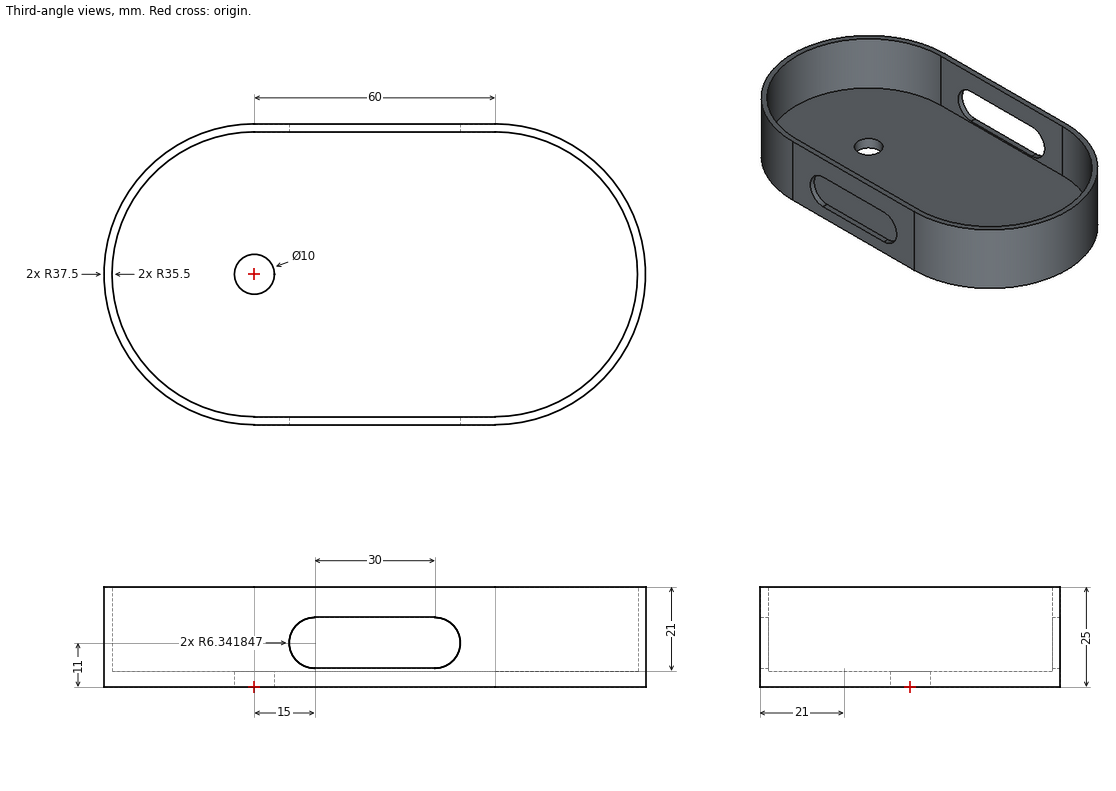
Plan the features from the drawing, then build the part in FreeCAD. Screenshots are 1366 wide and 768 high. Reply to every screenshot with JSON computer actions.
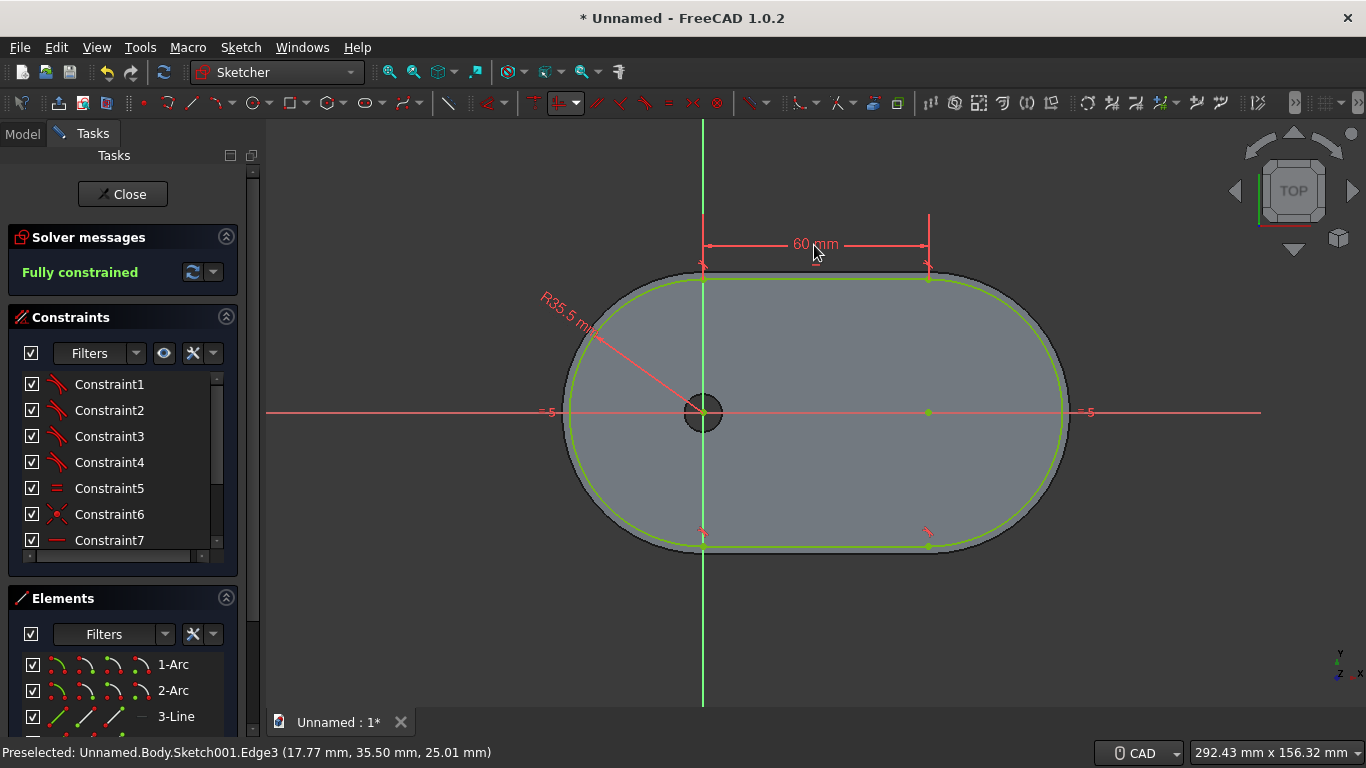
{"action": "left_click", "coordinate": [123, 194]}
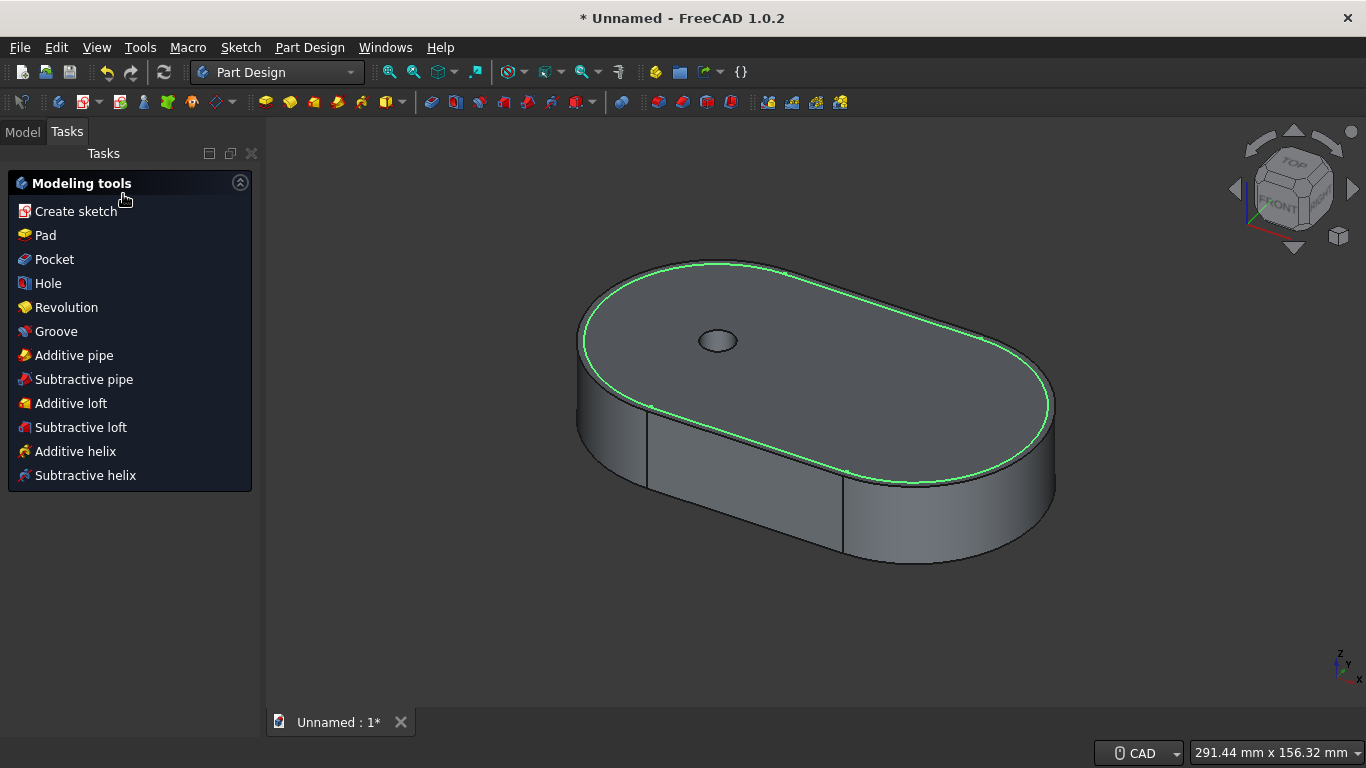
{"action": "left_click", "coordinate": [432, 102]}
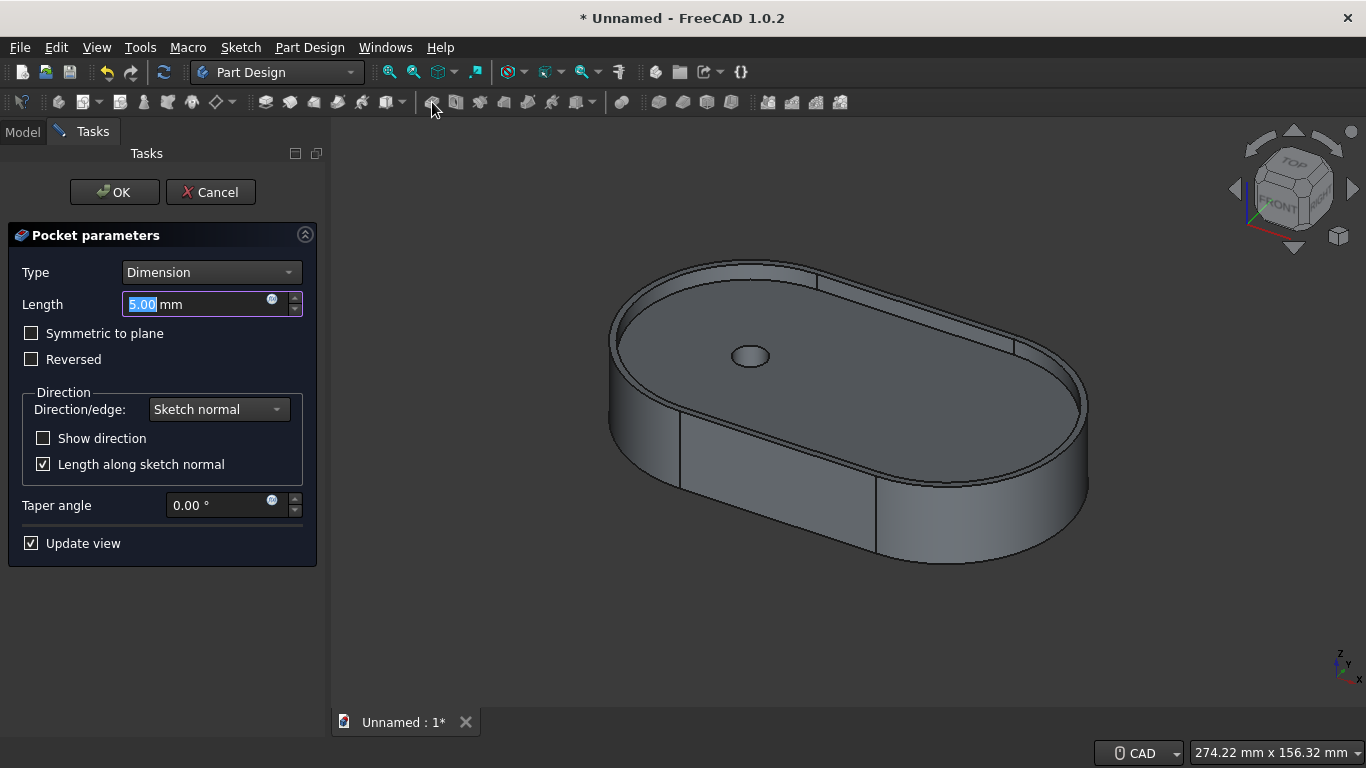
{"action": "type", "text": "21"}
{"action": "key", "text": "Tab"}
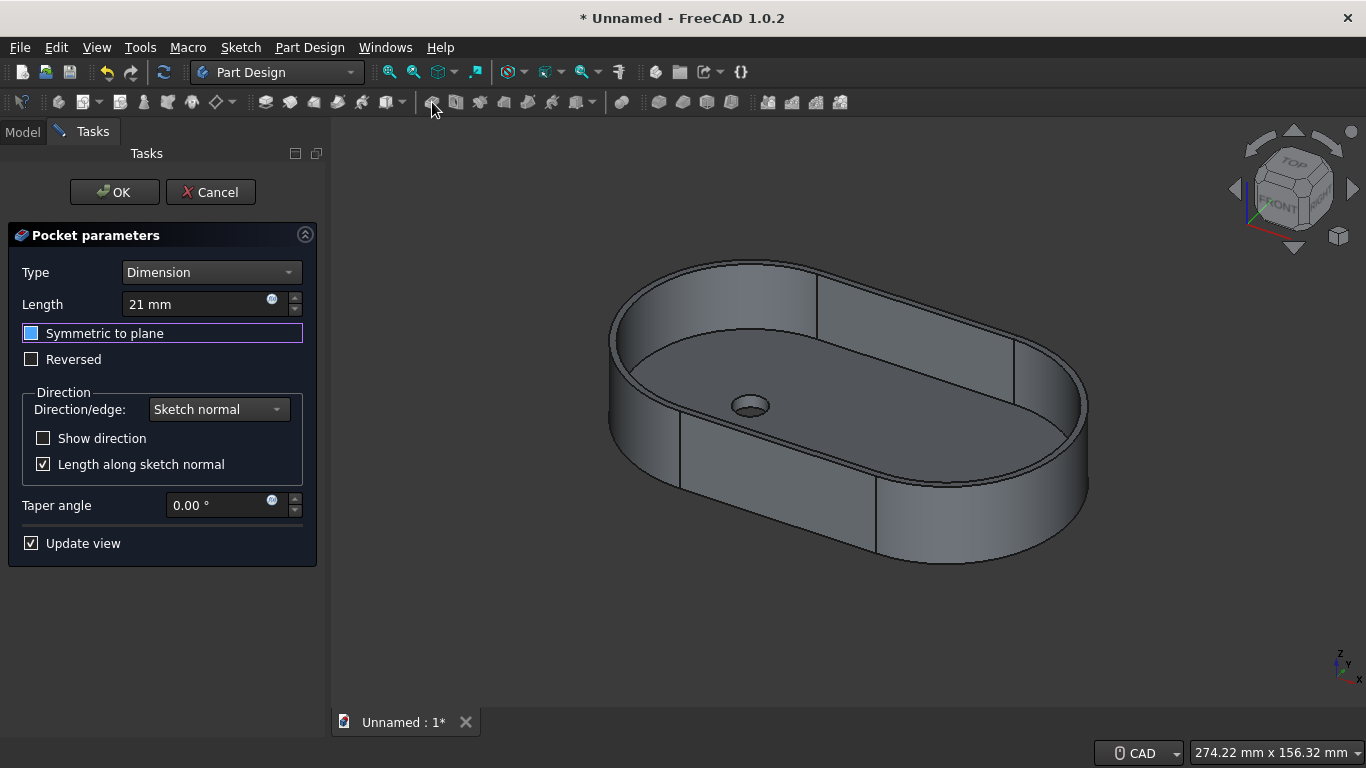
{"action": "left_click", "coordinate": [115, 192]}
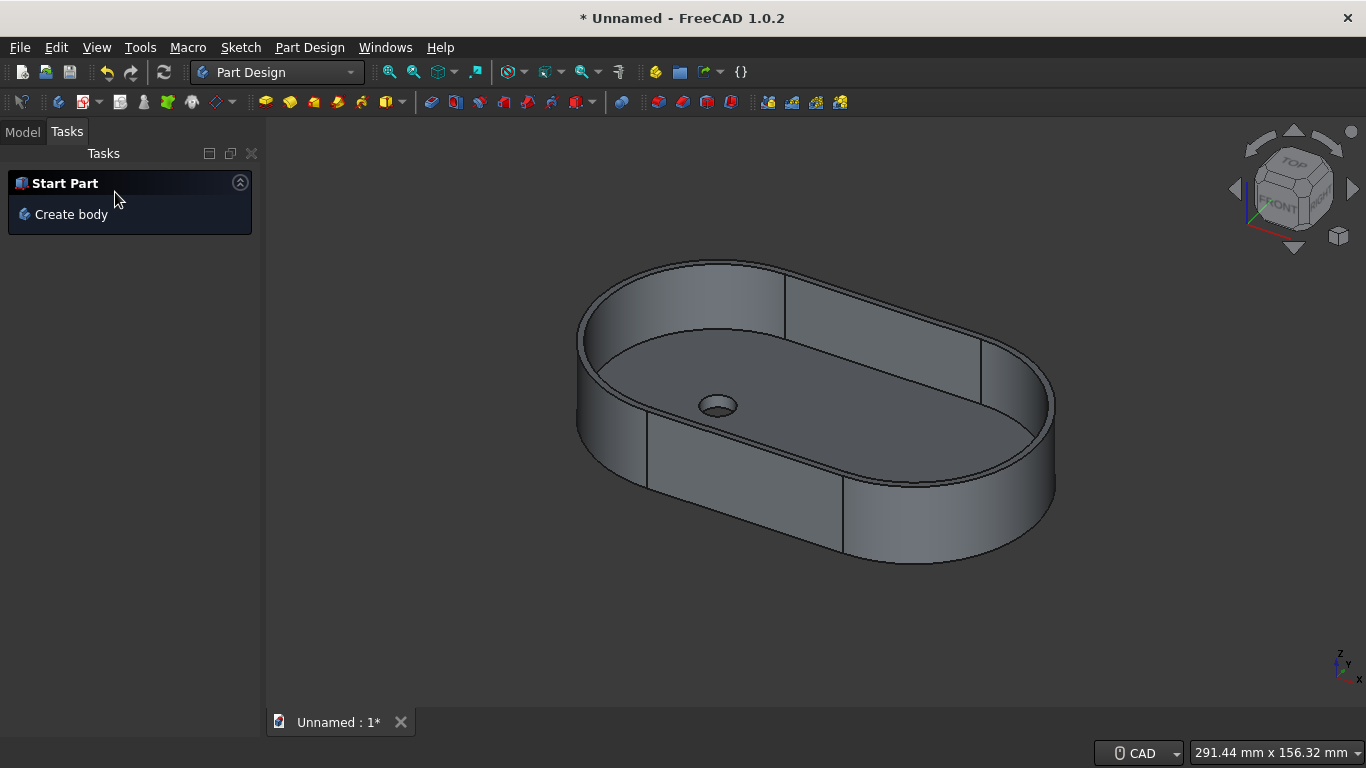
{"action": "left_click", "coordinate": [801, 500]}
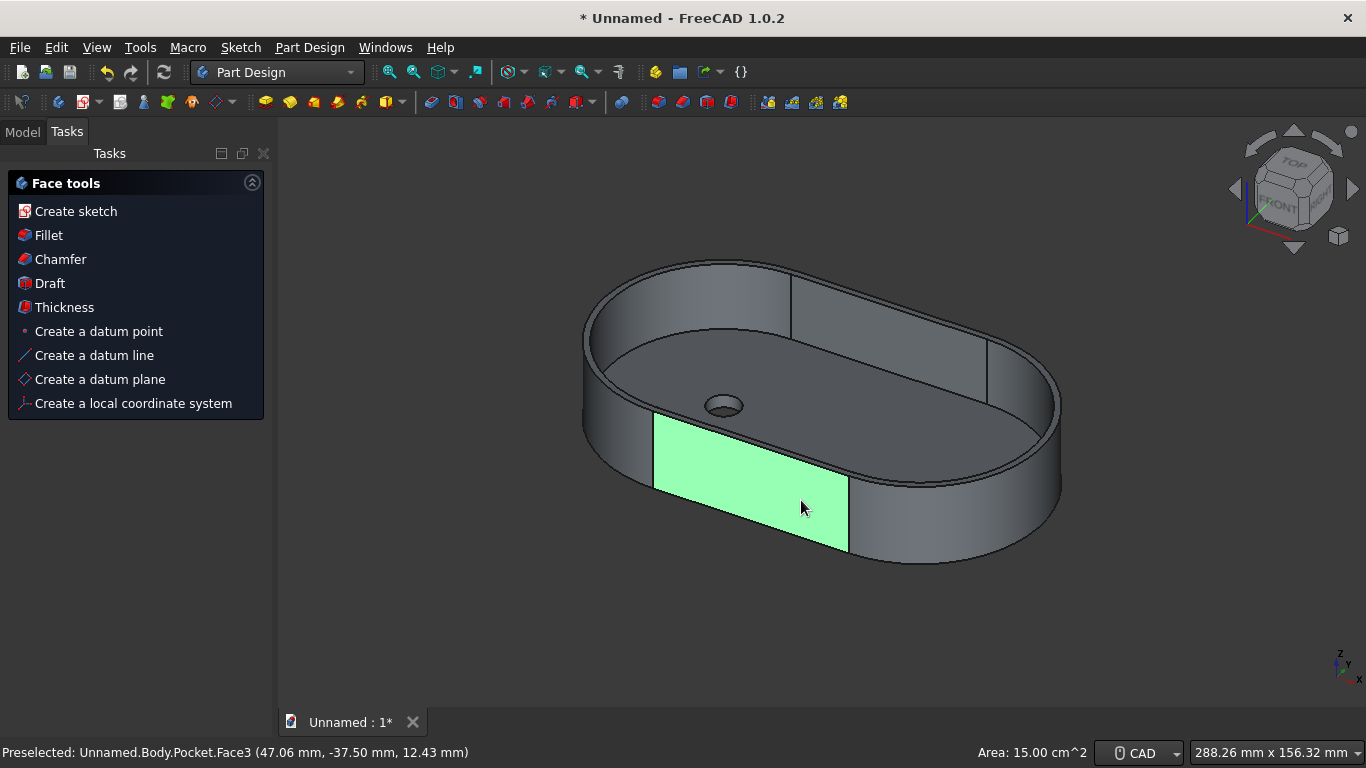
{"action": "left_click", "coordinate": [84, 102]}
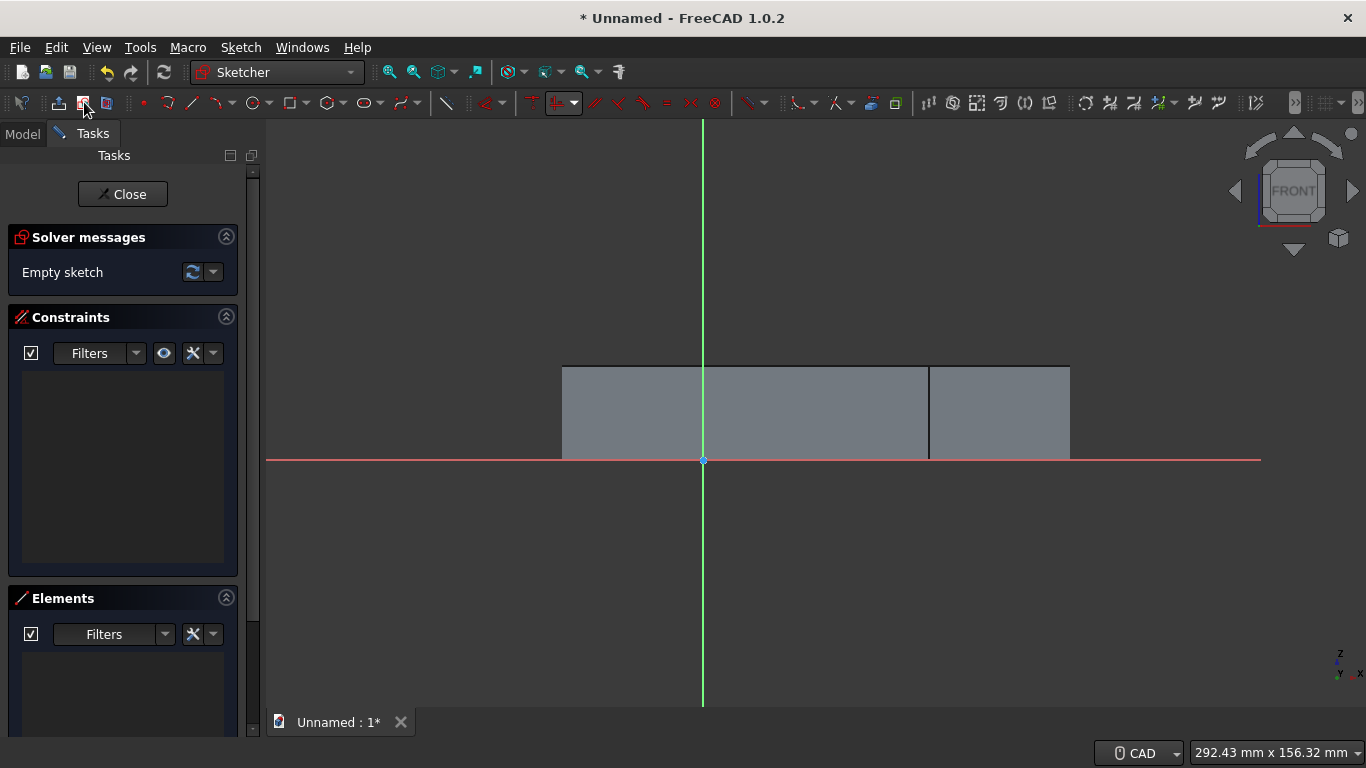
{"action": "scroll", "coordinate": [822, 434], "scroll_direction": "up", "scroll_amount": 6}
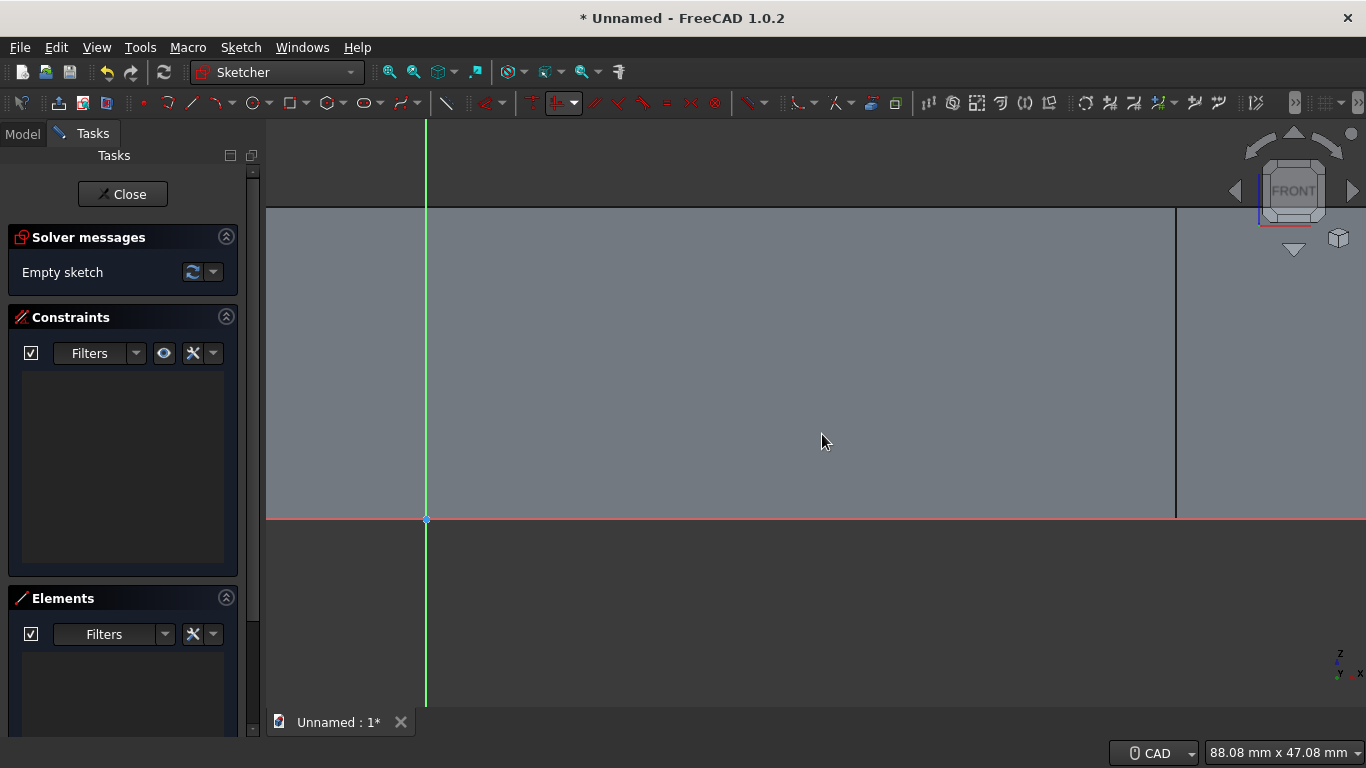
{"action": "left_click", "coordinate": [364, 104]}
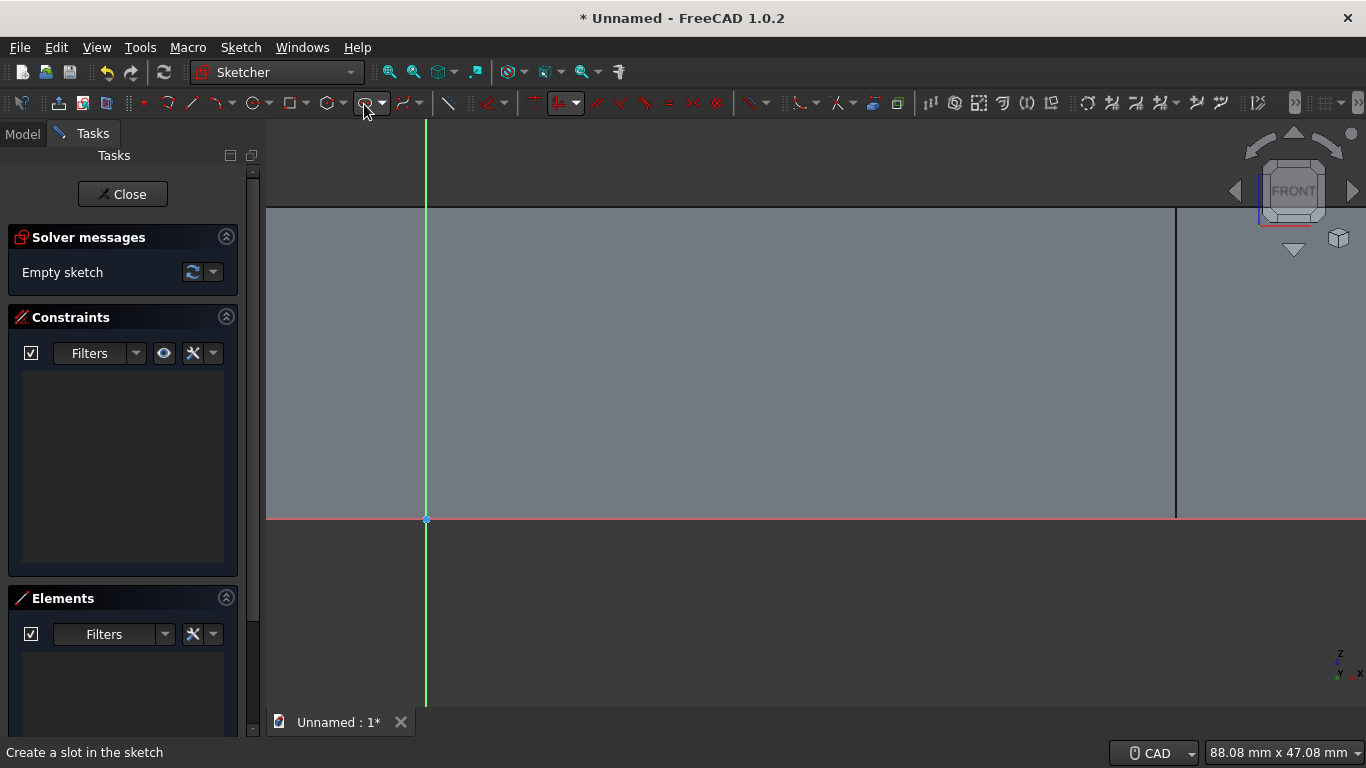
{"action": "left_click", "coordinate": [614, 382]}